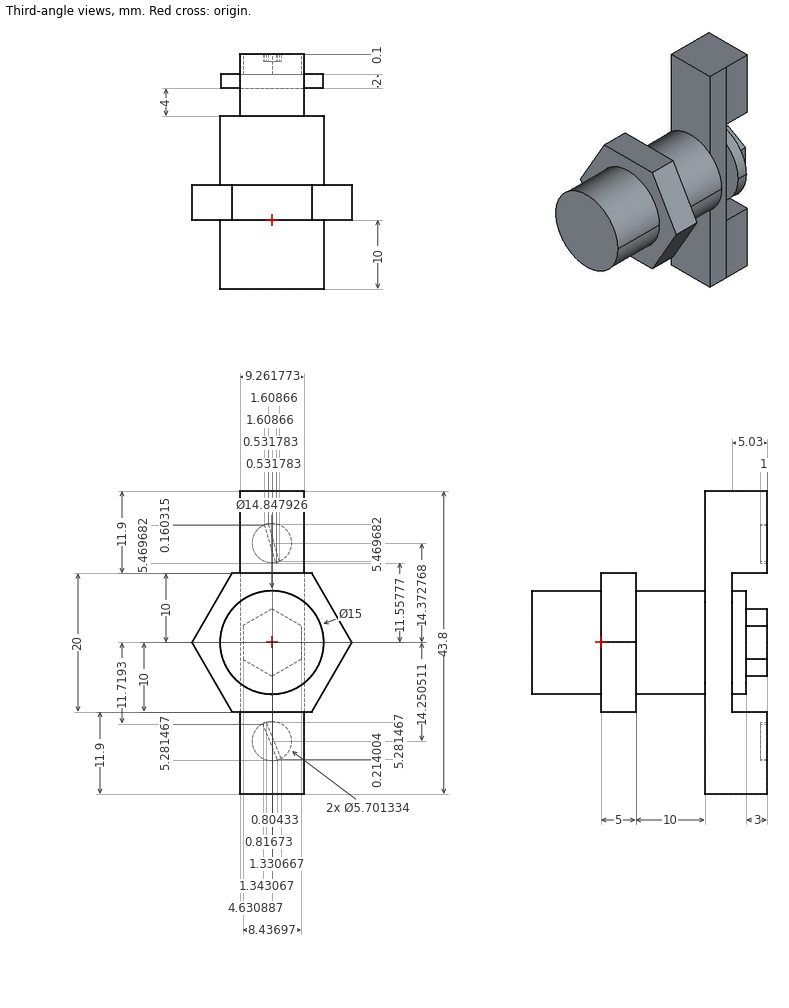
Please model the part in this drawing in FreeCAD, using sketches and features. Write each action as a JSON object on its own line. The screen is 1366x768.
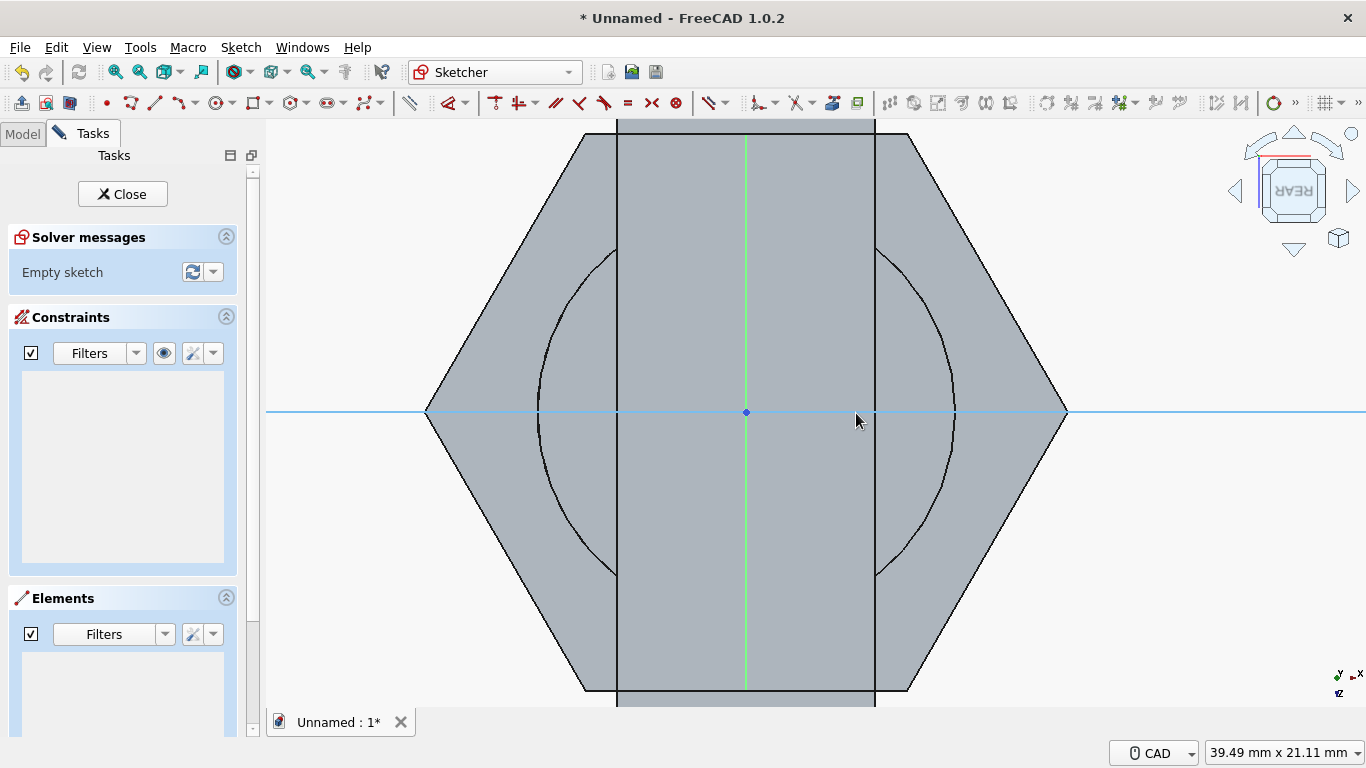
{"action": "left_click", "coordinate": [216, 104]}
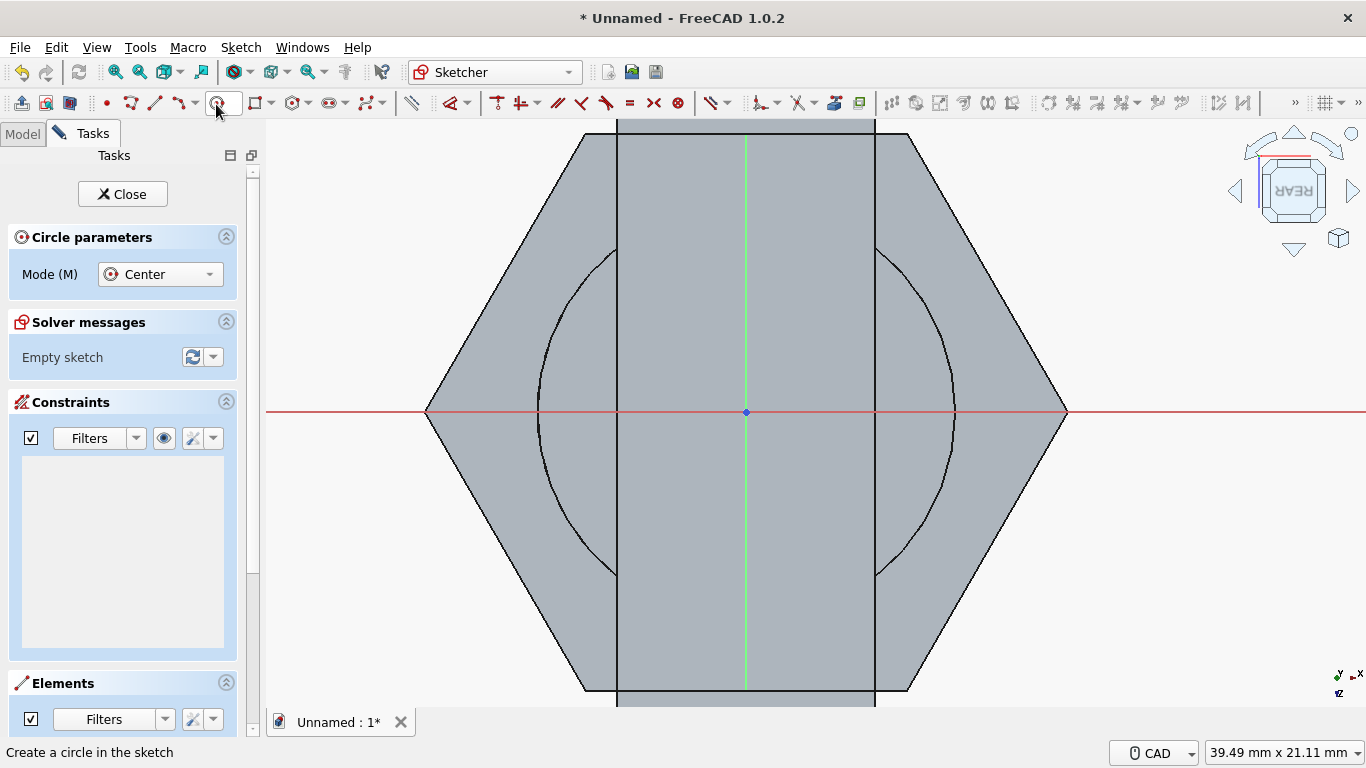
{"action": "left_click", "coordinate": [746, 412]}
{"action": "left_click", "coordinate": [893, 266]}
{"action": "key", "text": "Escape"}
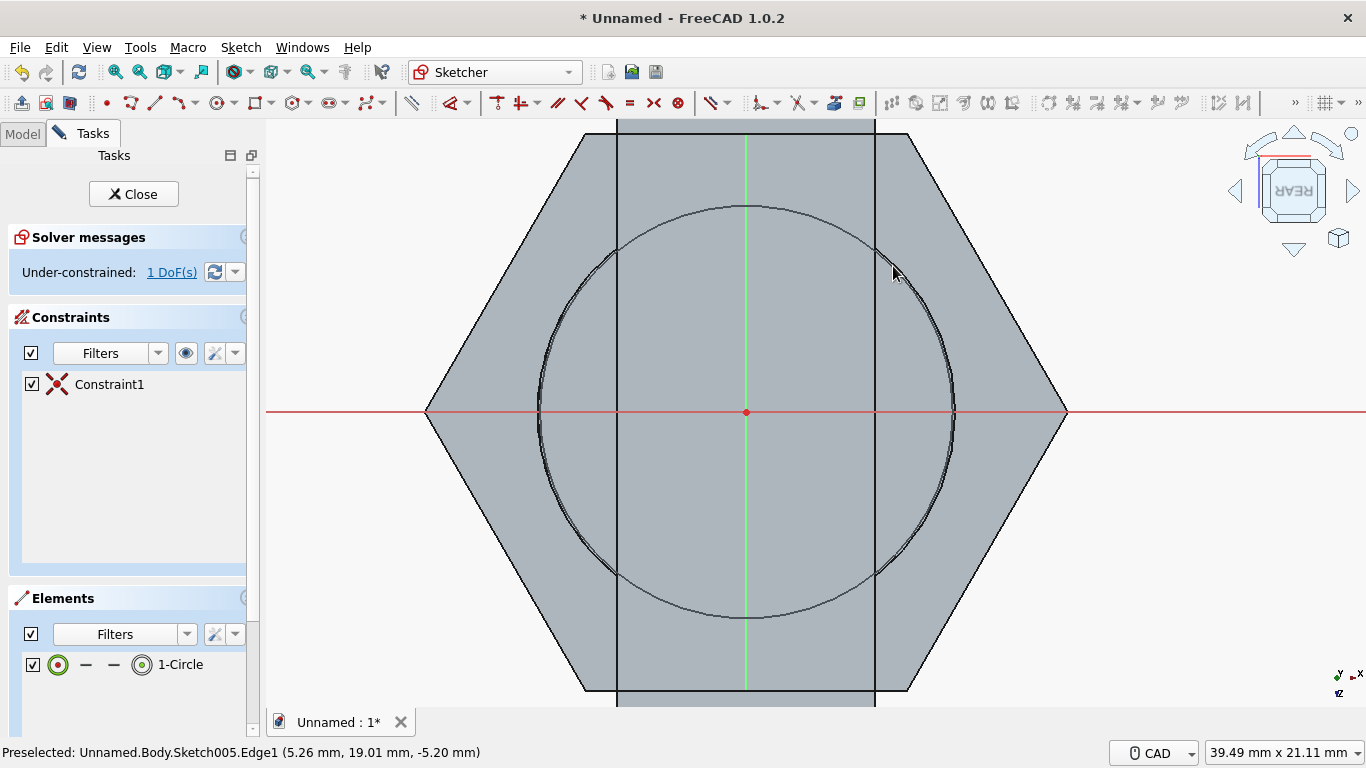
{"action": "left_click", "coordinate": [450, 104]}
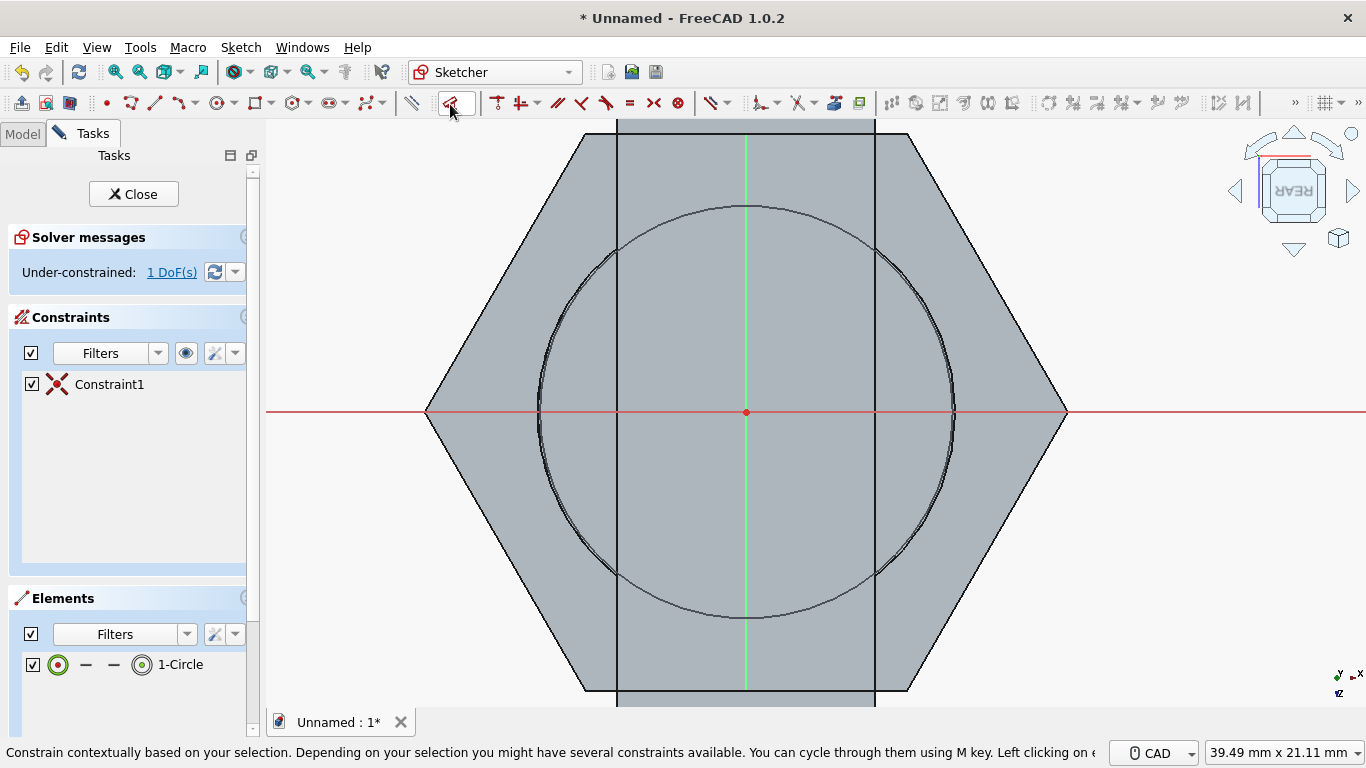
{"action": "left_click", "coordinate": [892, 266]}
{"action": "left_click", "coordinate": [915, 243]}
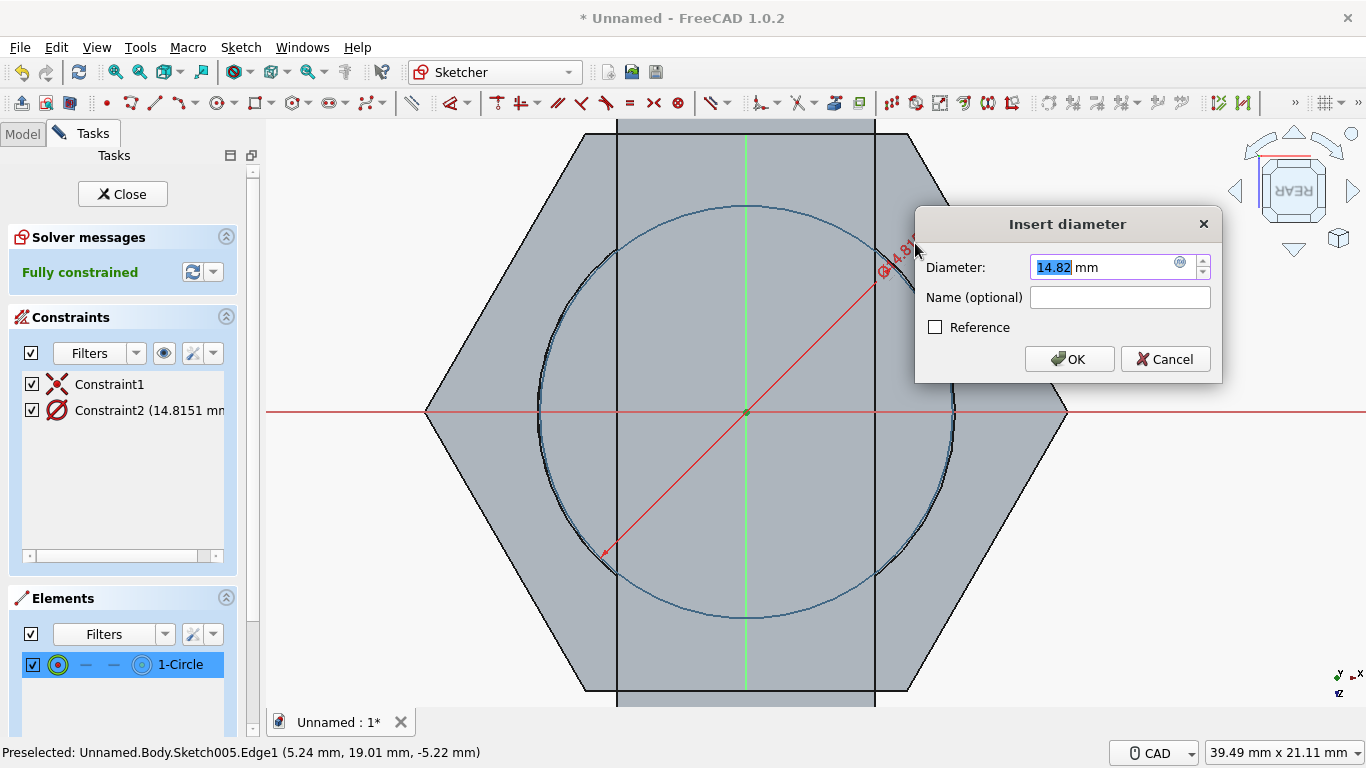
{"action": "type", "text": "14.847926"}
{"action": "key", "text": "Return"}
{"action": "key", "text": "Escape"}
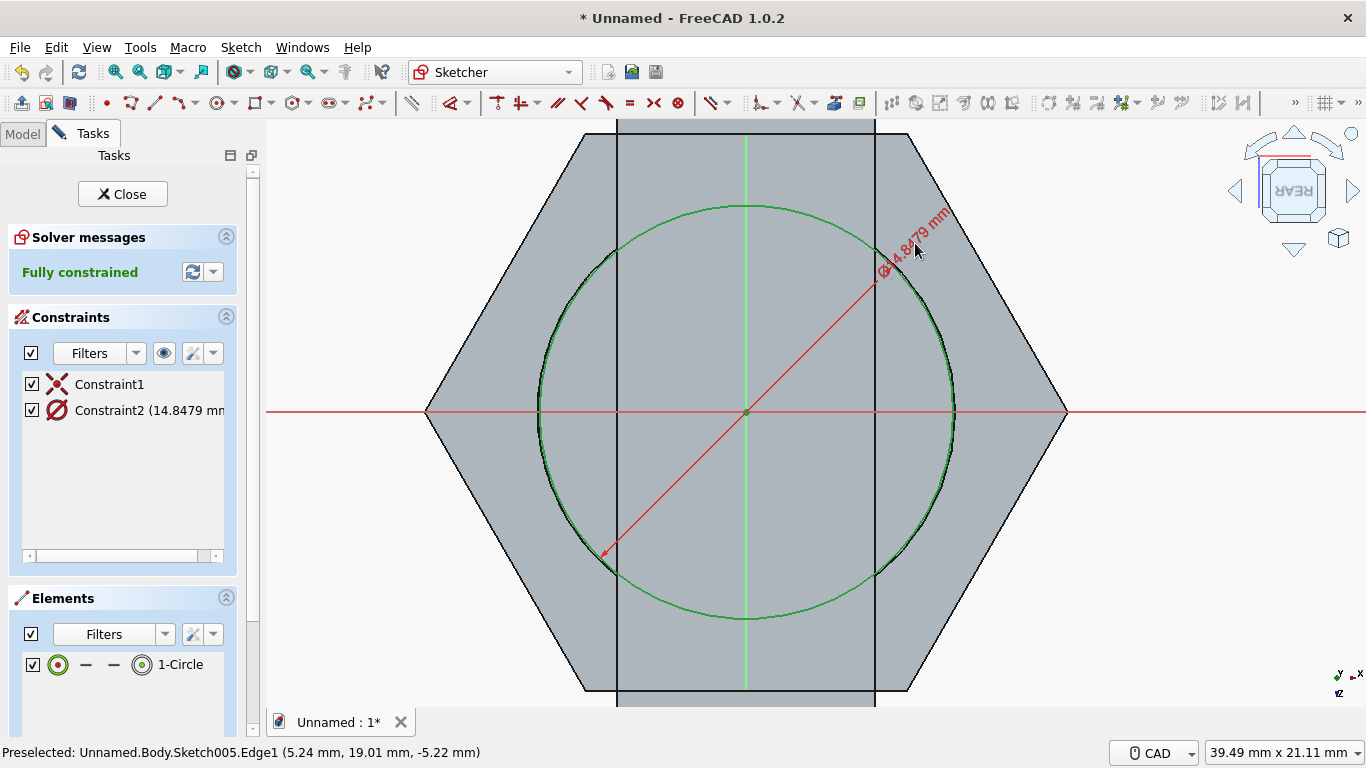
{"action": "left_click", "coordinate": [123, 194]}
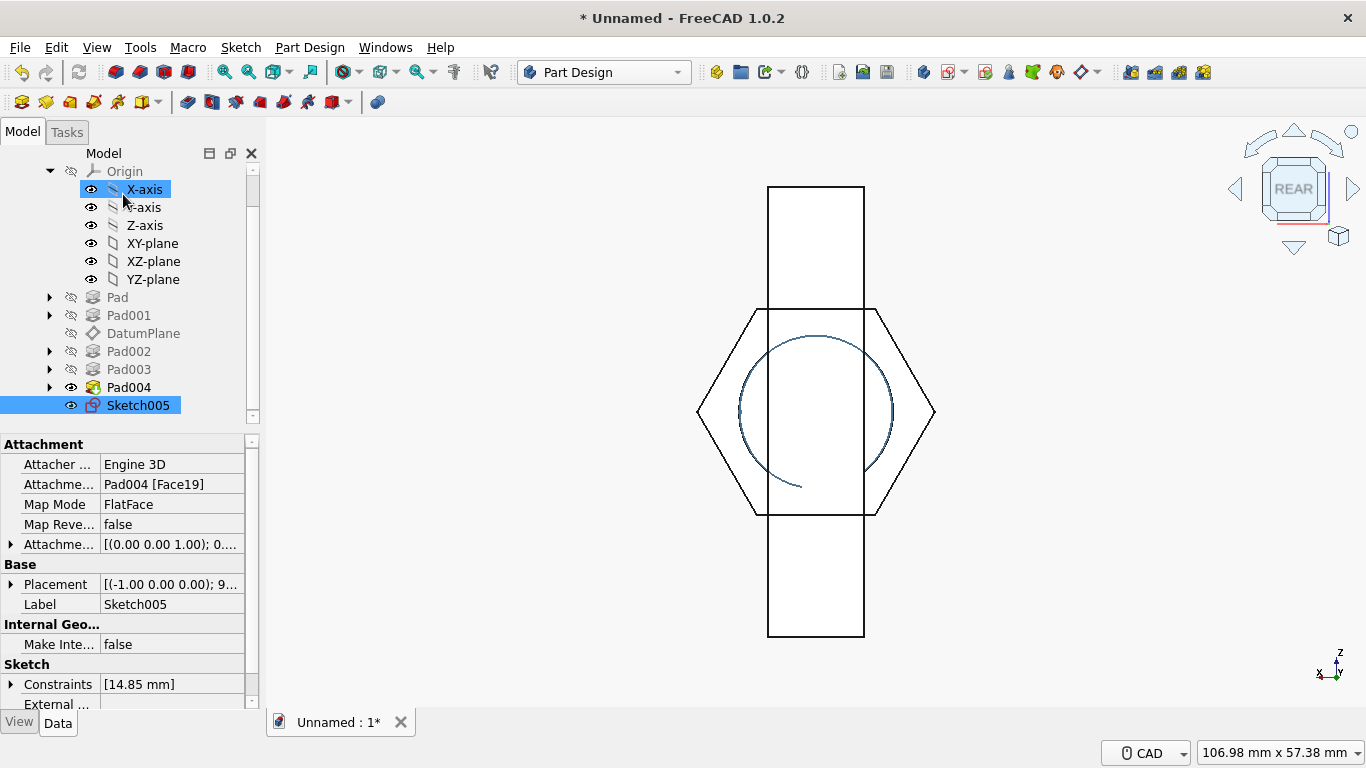
{"action": "left_click", "coordinate": [22, 102]}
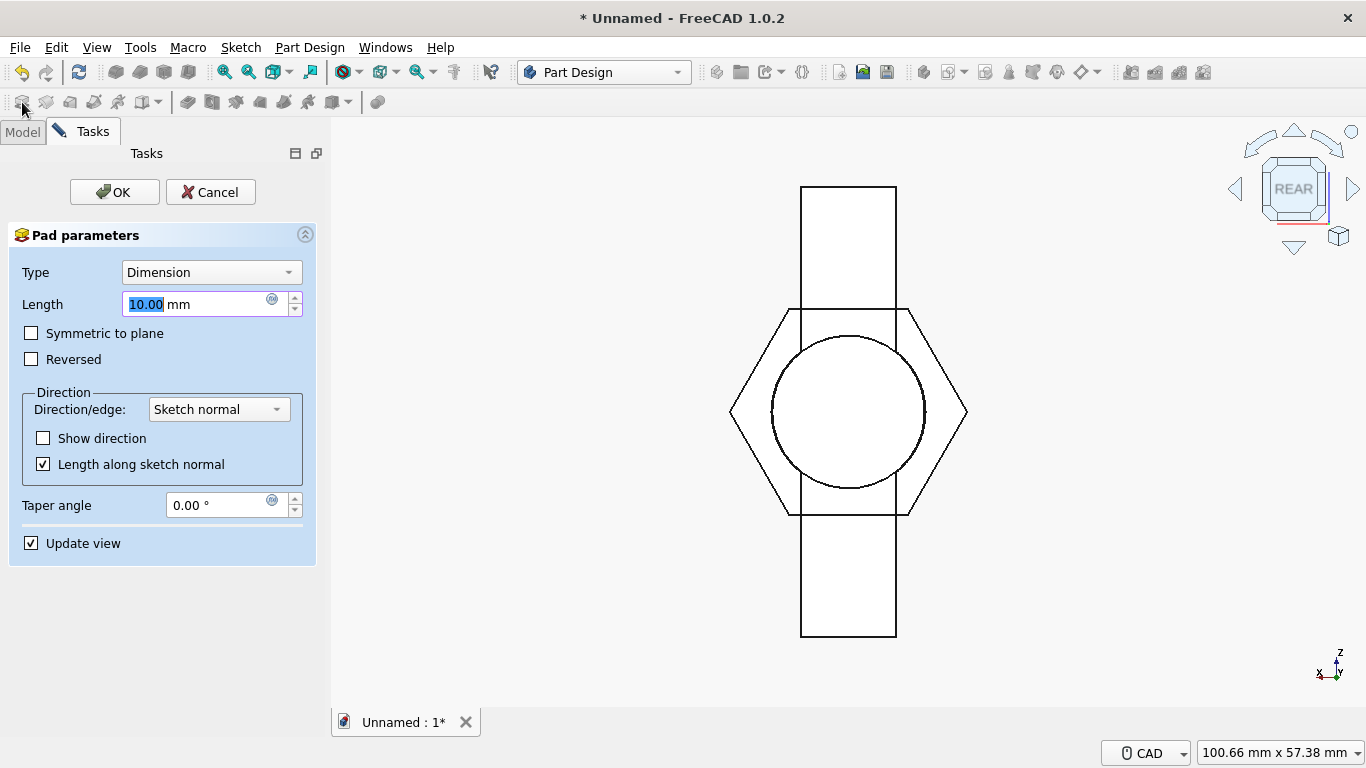
{"action": "type", "text": "2"}
{"action": "key", "text": "Tab"}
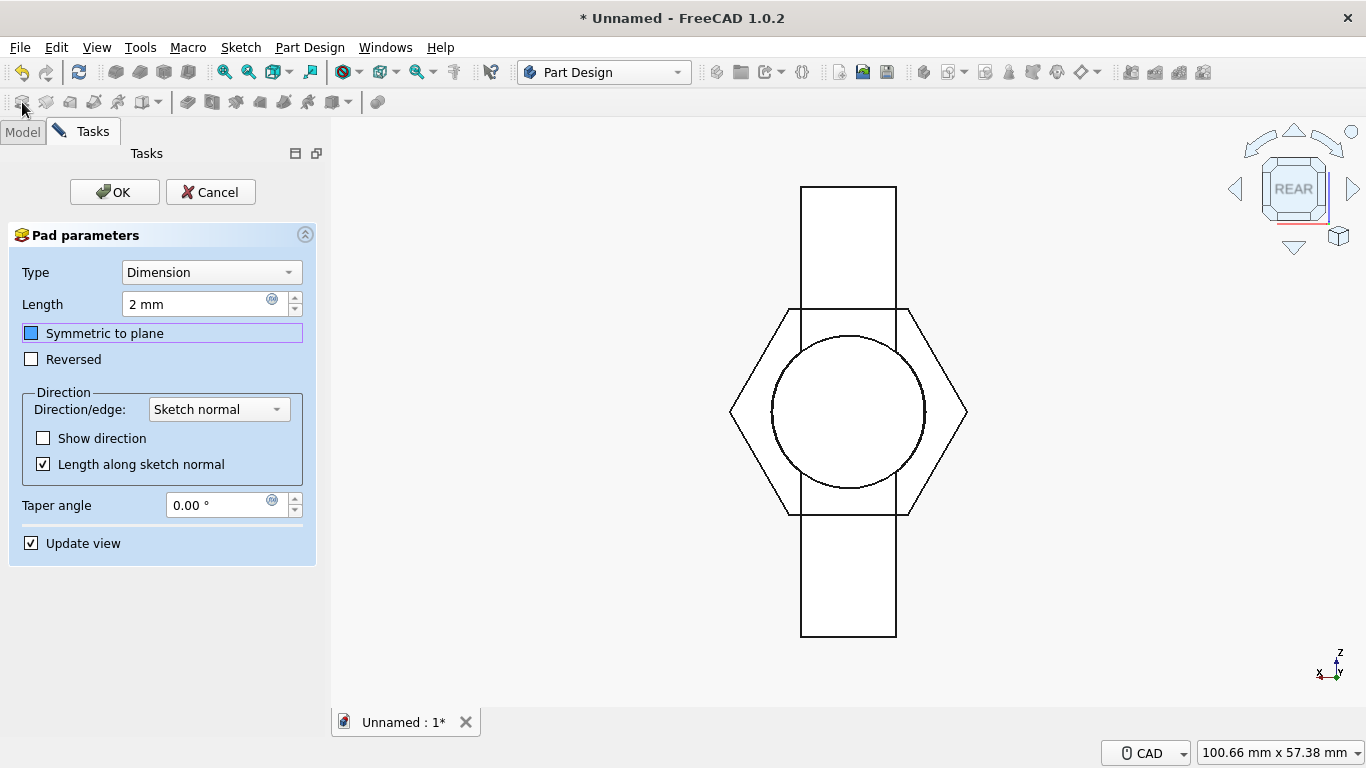
{"action": "left_click", "coordinate": [115, 192]}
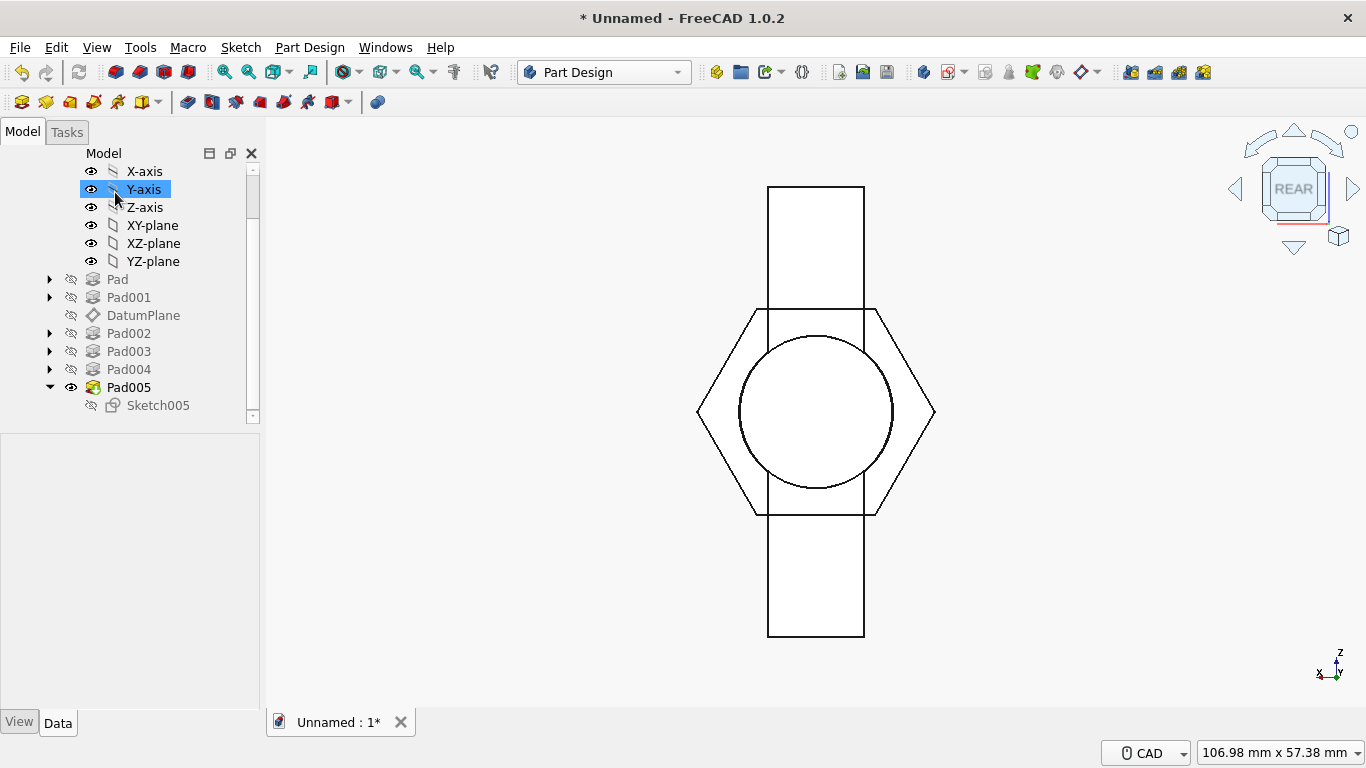
{"action": "left_click", "coordinate": [816, 411]}